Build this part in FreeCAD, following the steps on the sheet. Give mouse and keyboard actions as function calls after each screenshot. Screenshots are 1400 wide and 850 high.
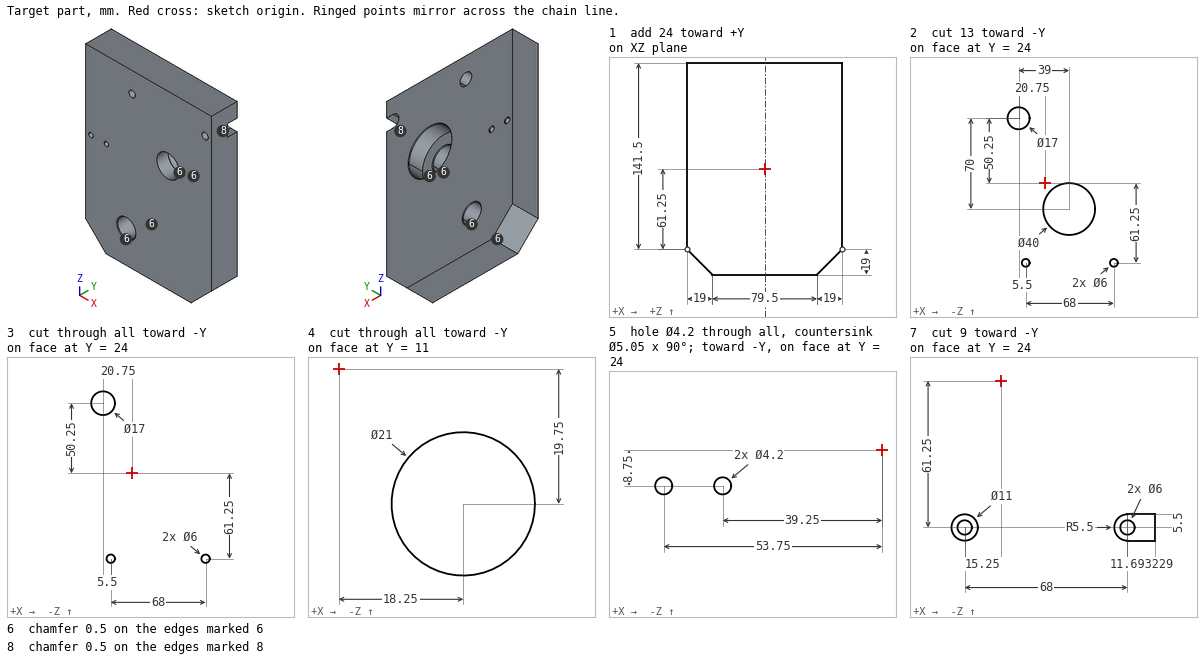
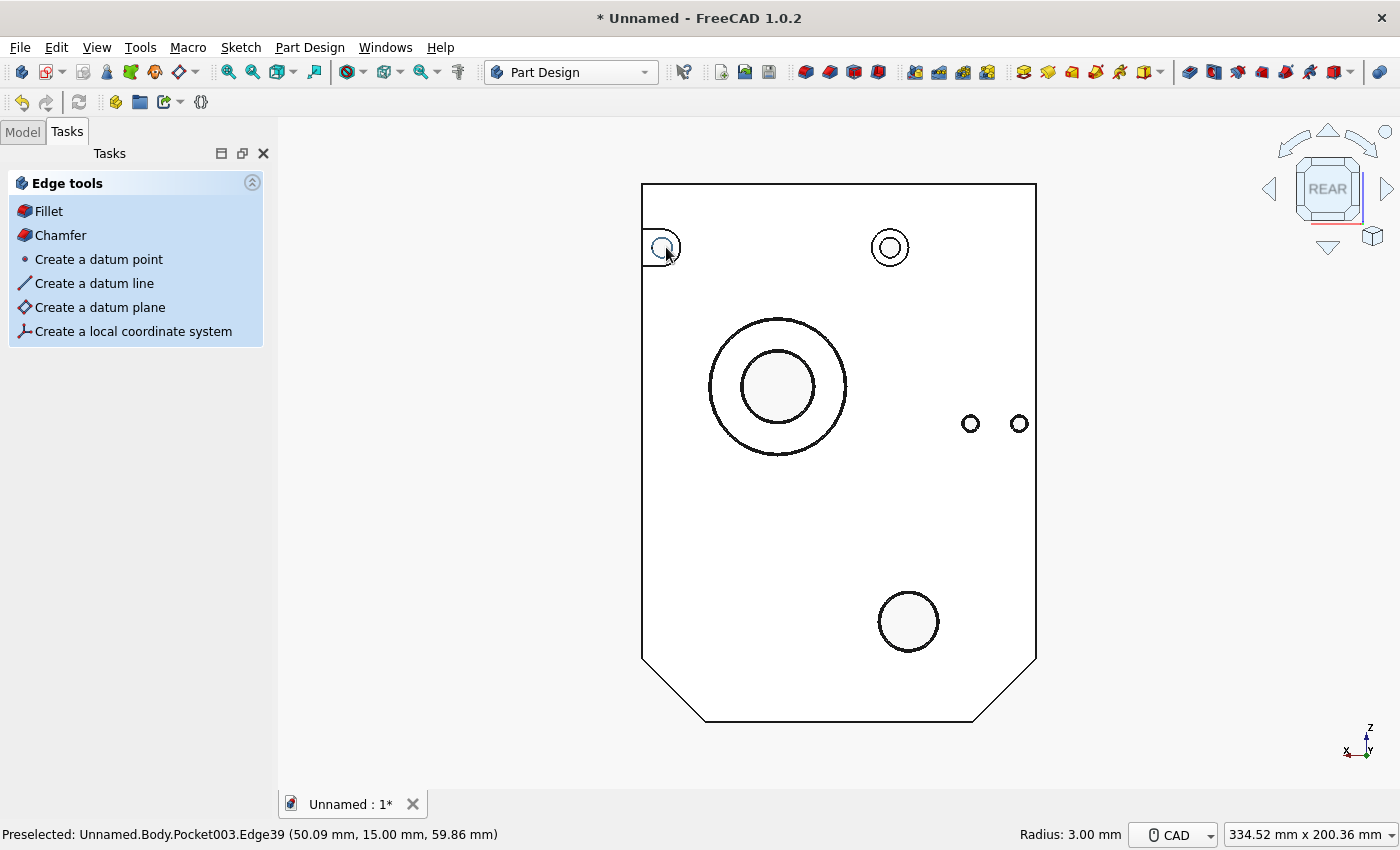
click(830, 72)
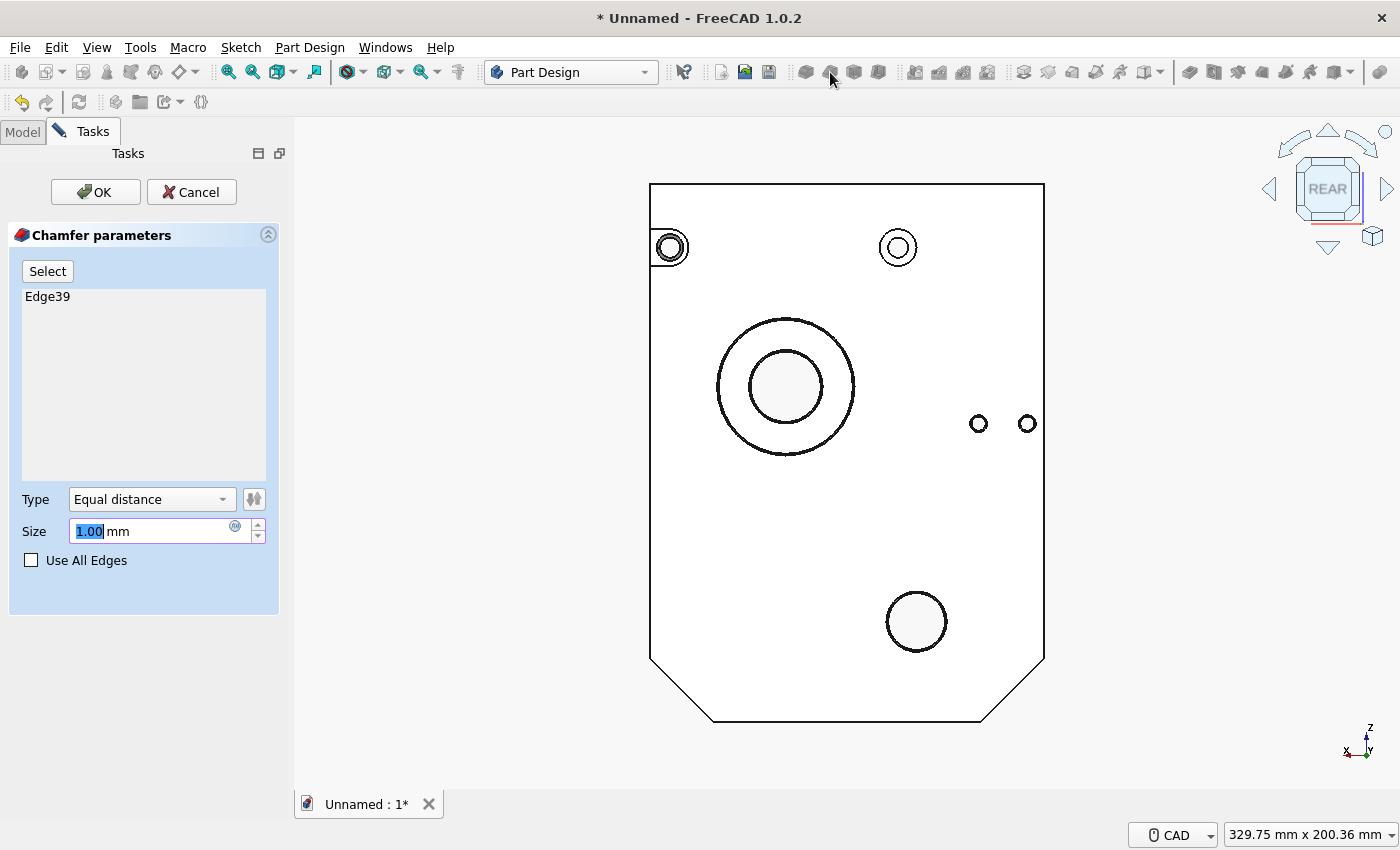
text(0.5)
key(Tab)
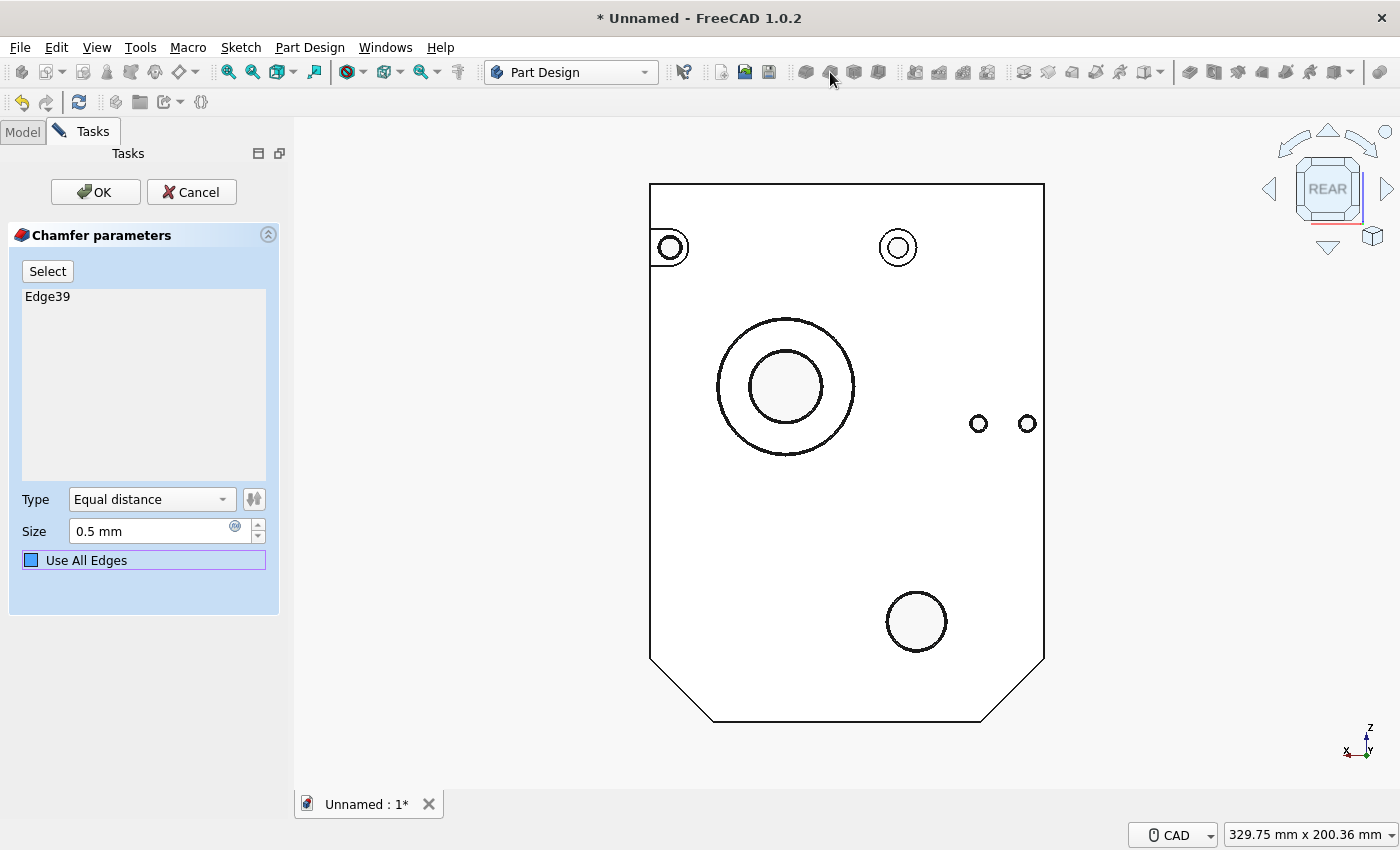
click(96, 192)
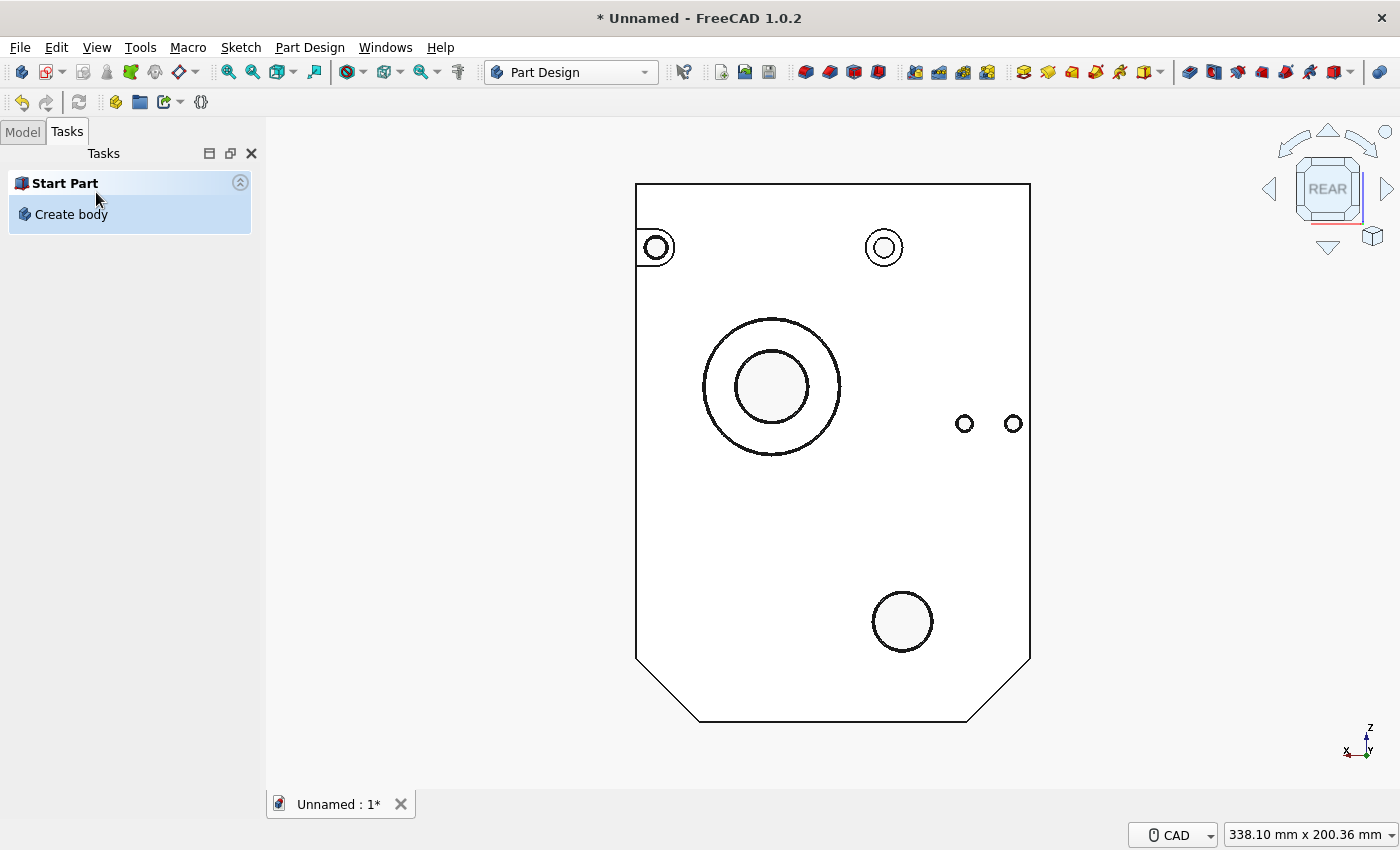
key(0)